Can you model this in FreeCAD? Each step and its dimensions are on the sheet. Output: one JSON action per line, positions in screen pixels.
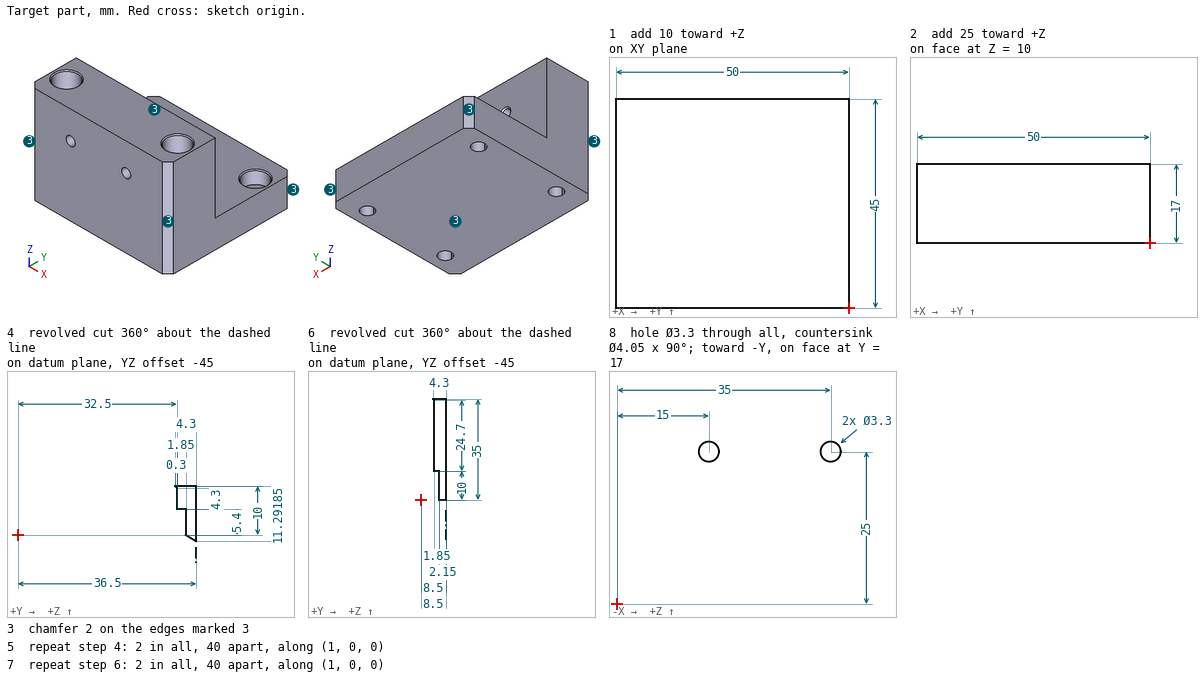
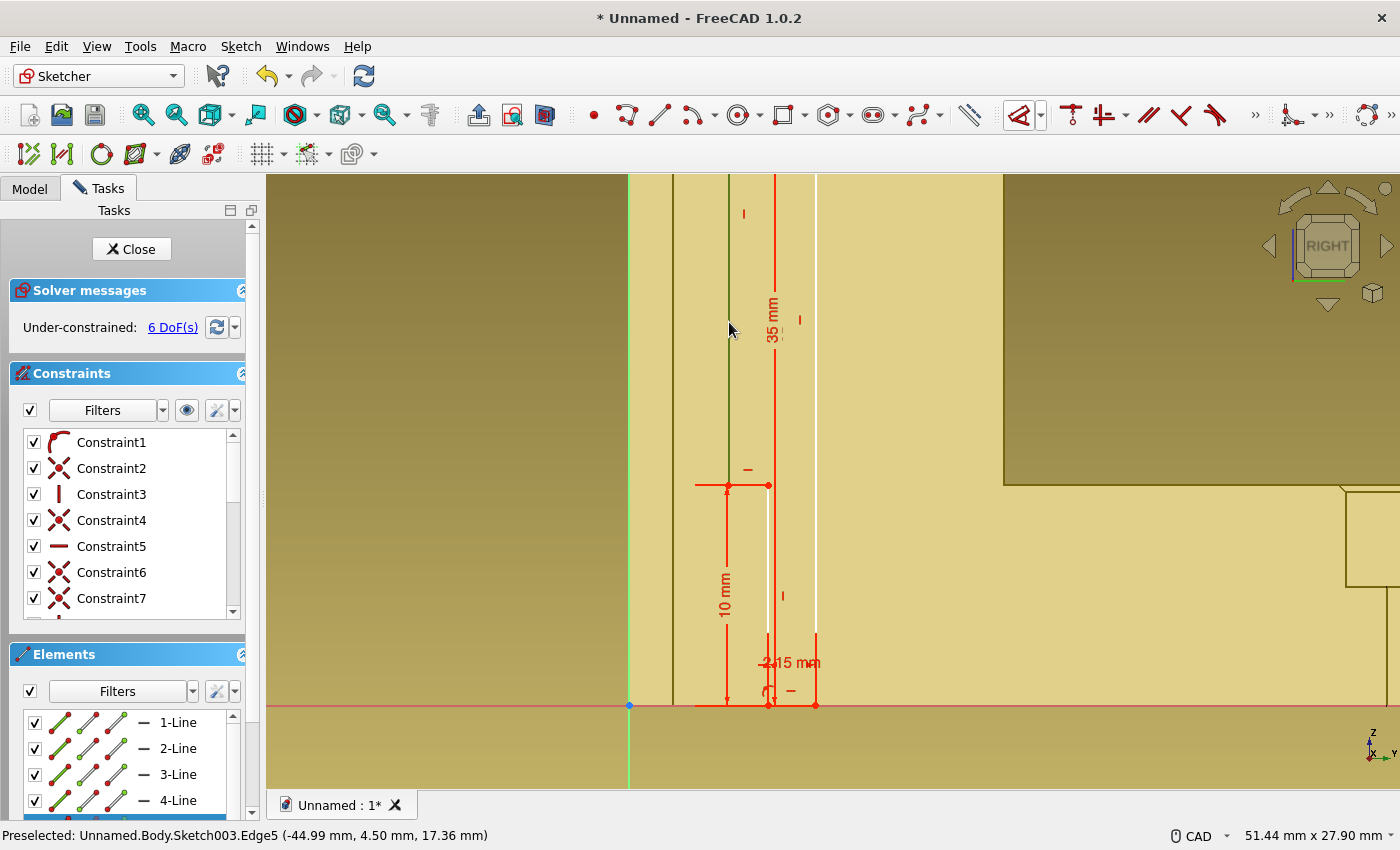
{"action": "key", "text": "i"}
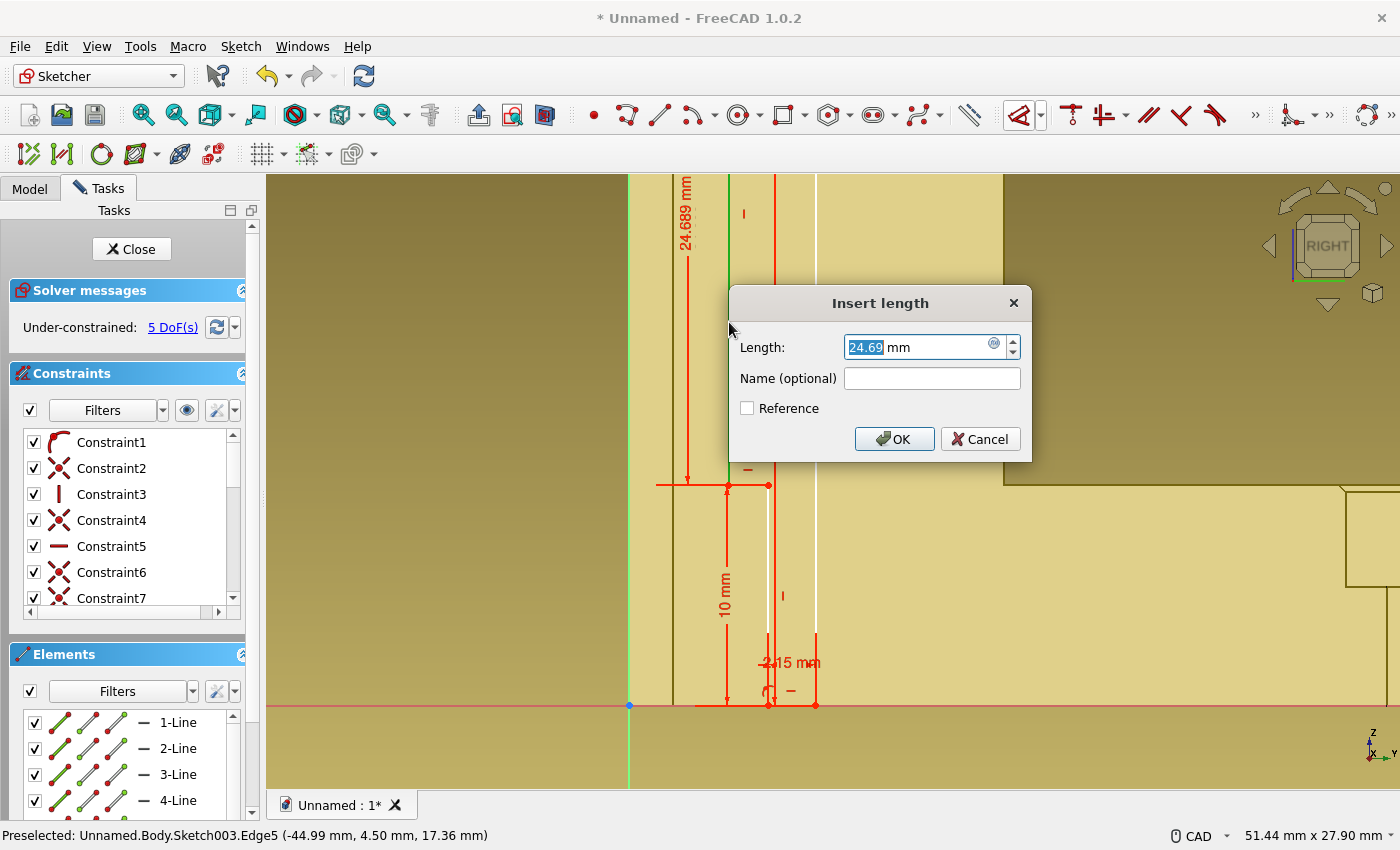
{"action": "type", "text": "24.7"}
{"action": "key", "text": "Return"}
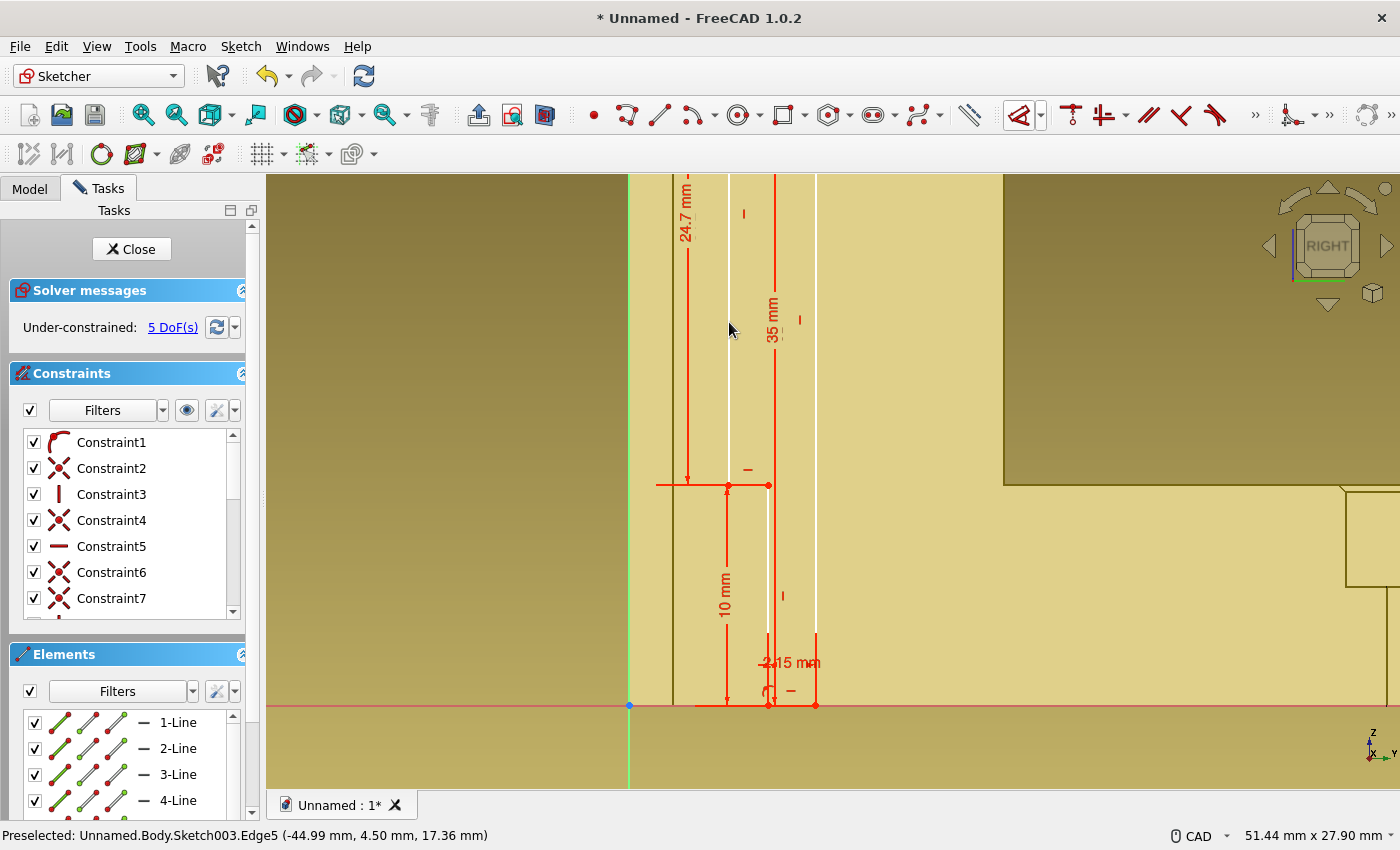
{"action": "left_click", "coordinate": [741, 485]}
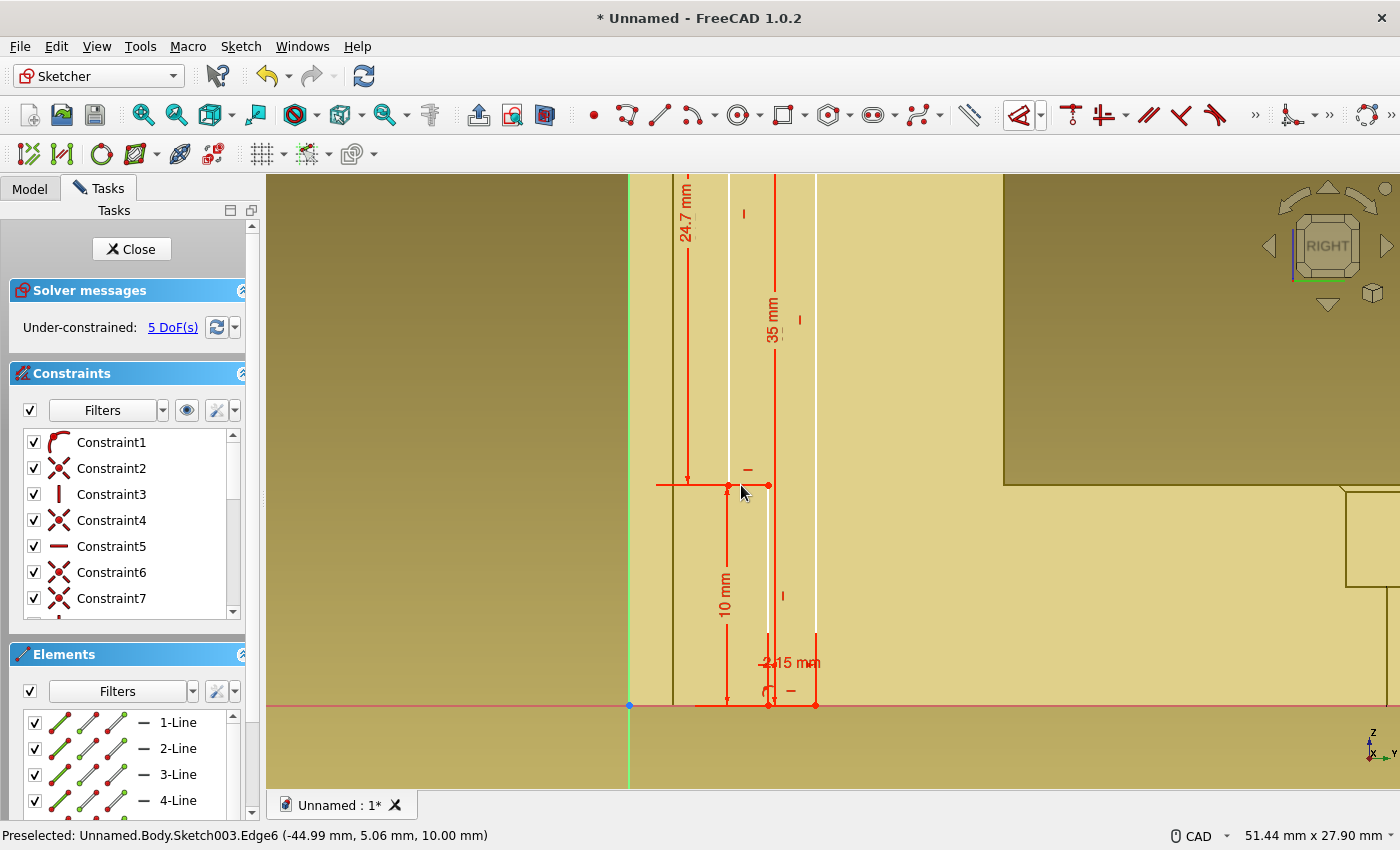
{"action": "key", "text": "l"}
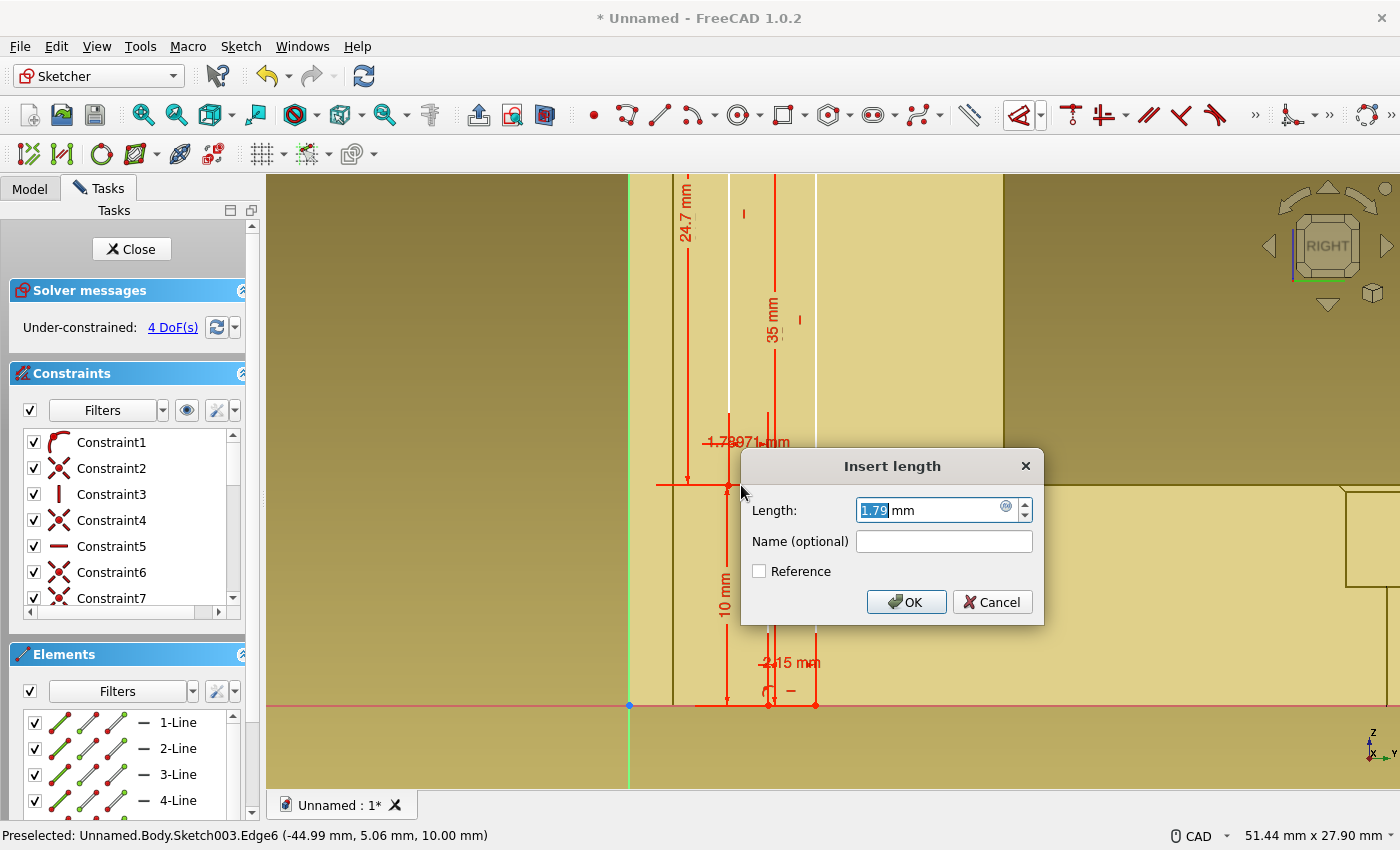
{"action": "type", "text": "1.85"}
{"action": "key", "text": "Return"}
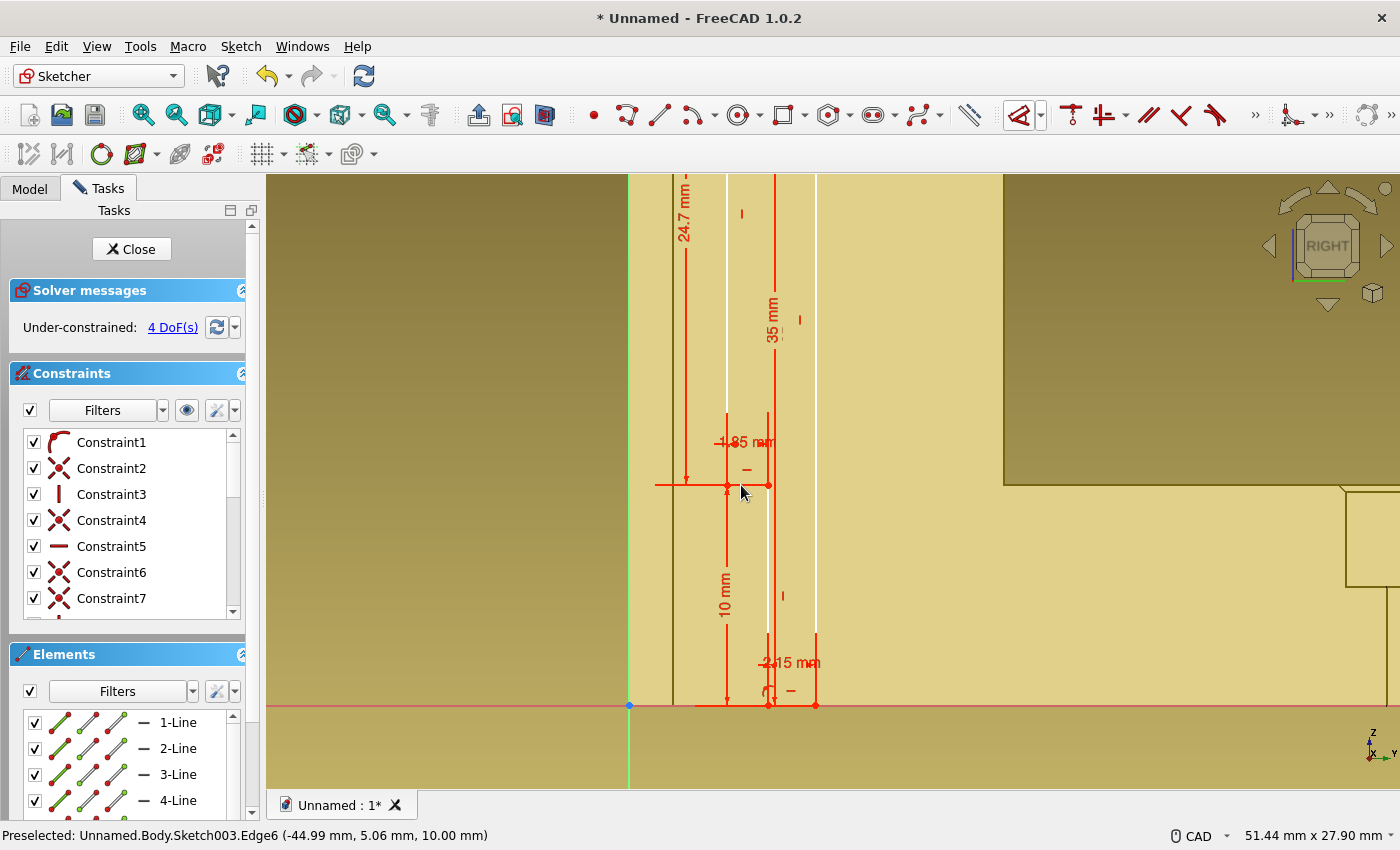
{"action": "left_click", "coordinate": [816, 706]}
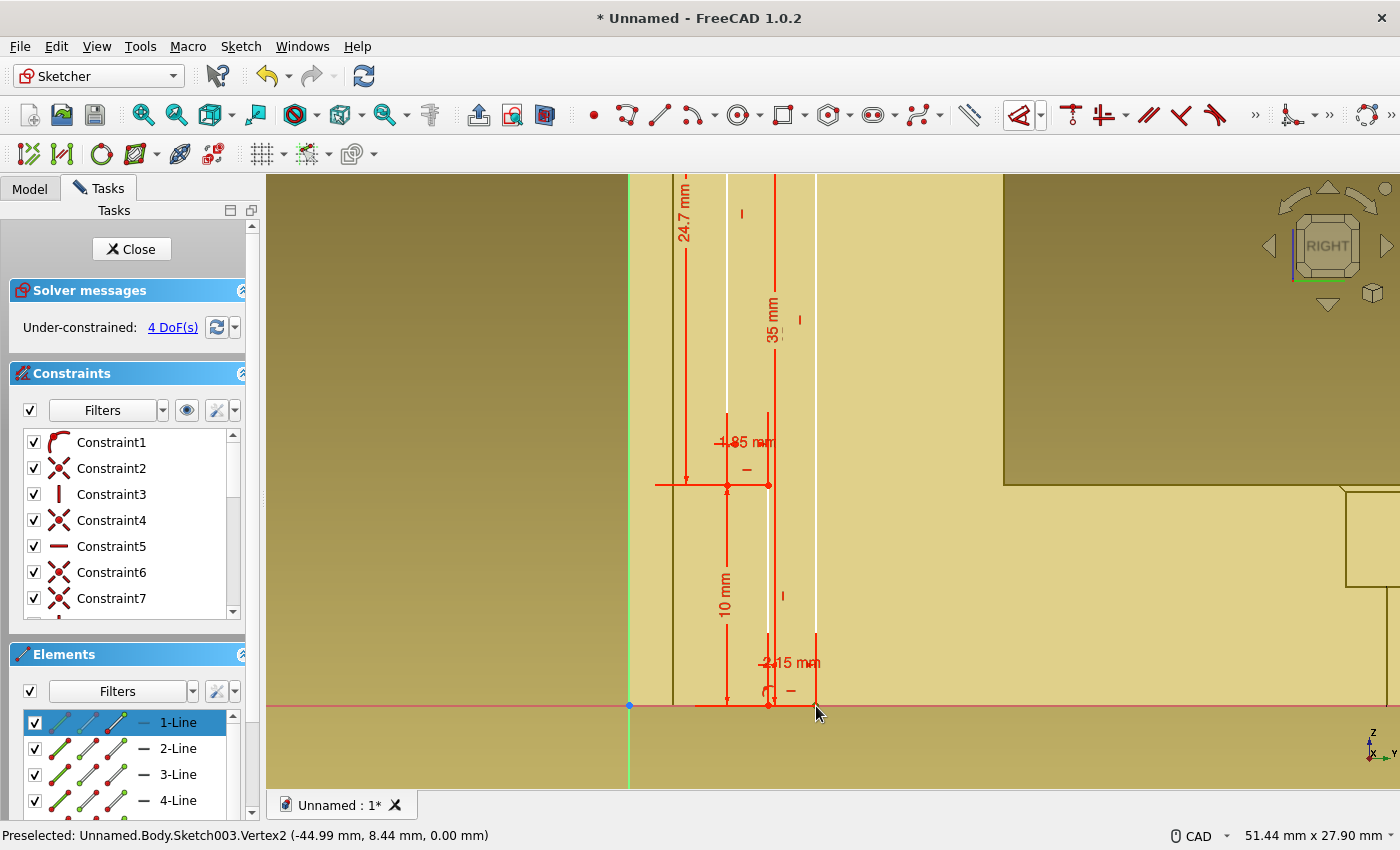
{"action": "key", "text": "l"}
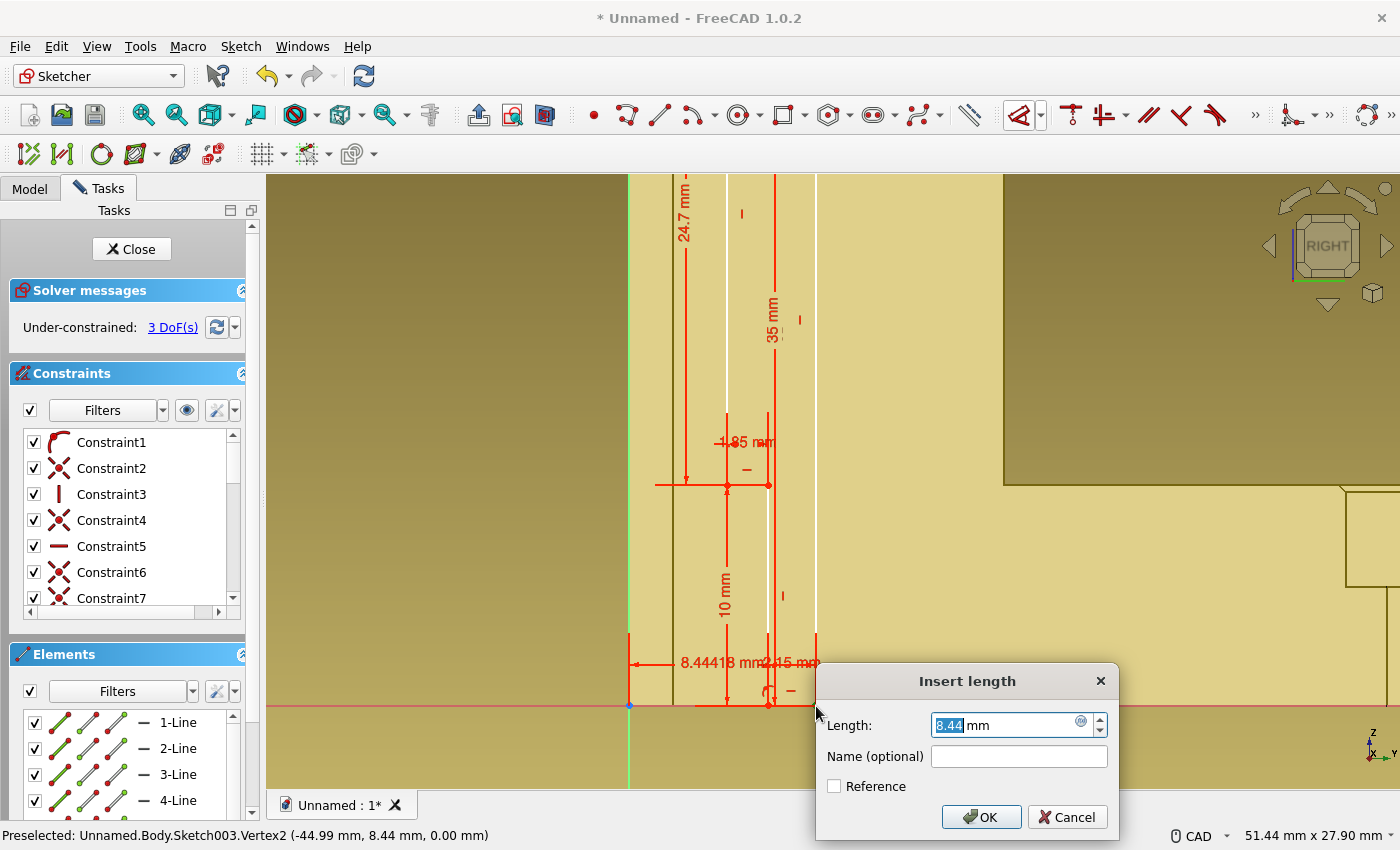
{"action": "type", "text": "8.5"}
{"action": "key", "text": "Return"}